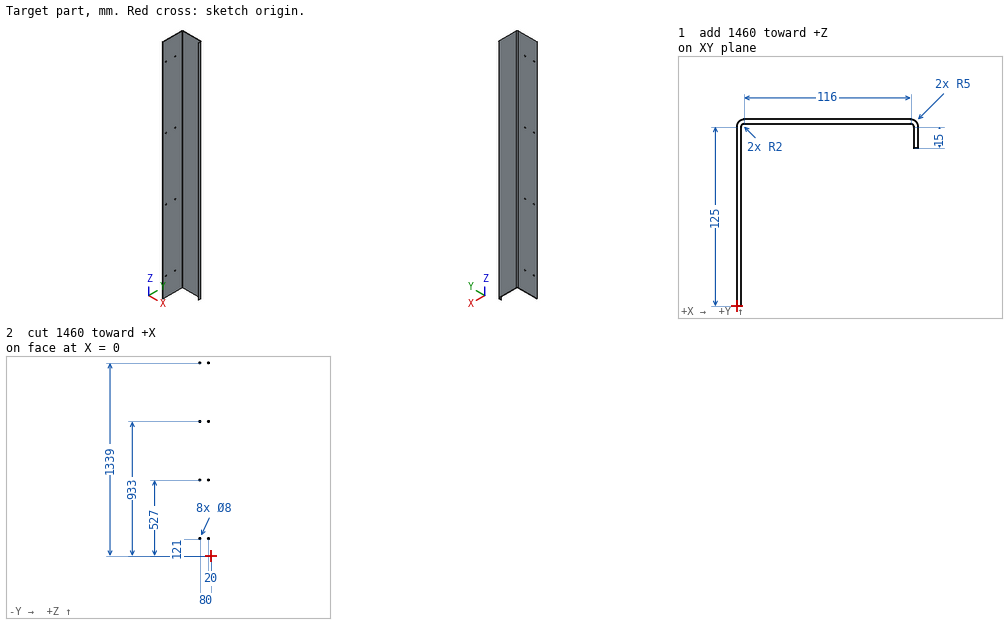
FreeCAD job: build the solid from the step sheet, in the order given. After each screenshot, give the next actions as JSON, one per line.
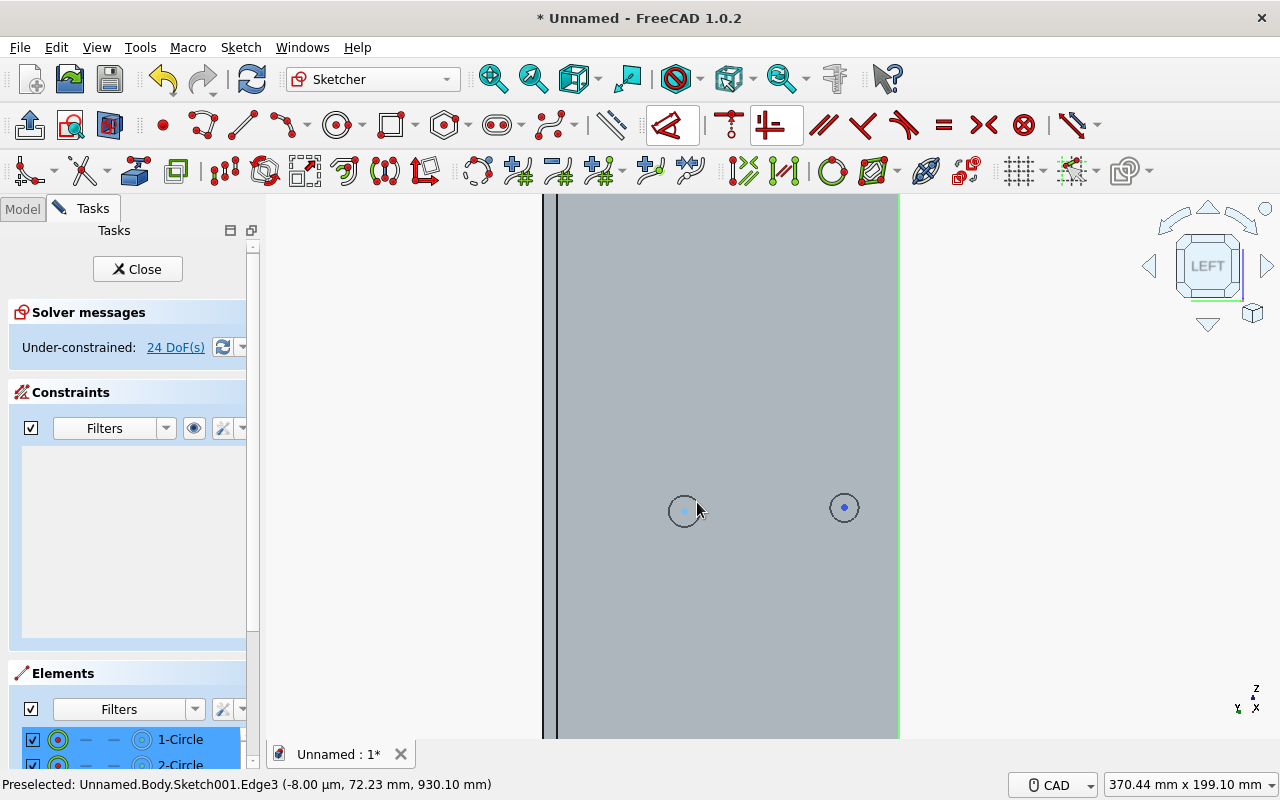
{"action": "left_click", "coordinate": [696, 500]}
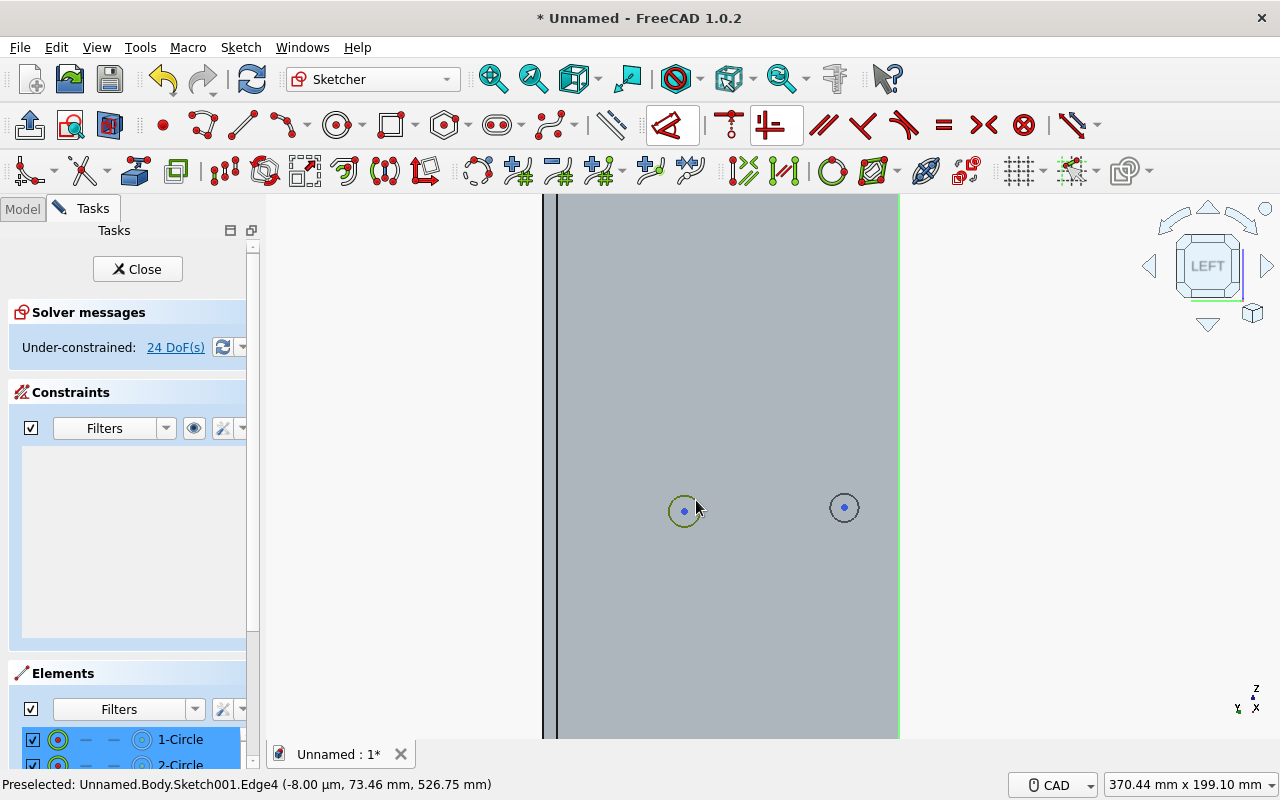
{"action": "scroll", "coordinate": [697, 502], "scroll_direction": "down", "scroll_amount": 12}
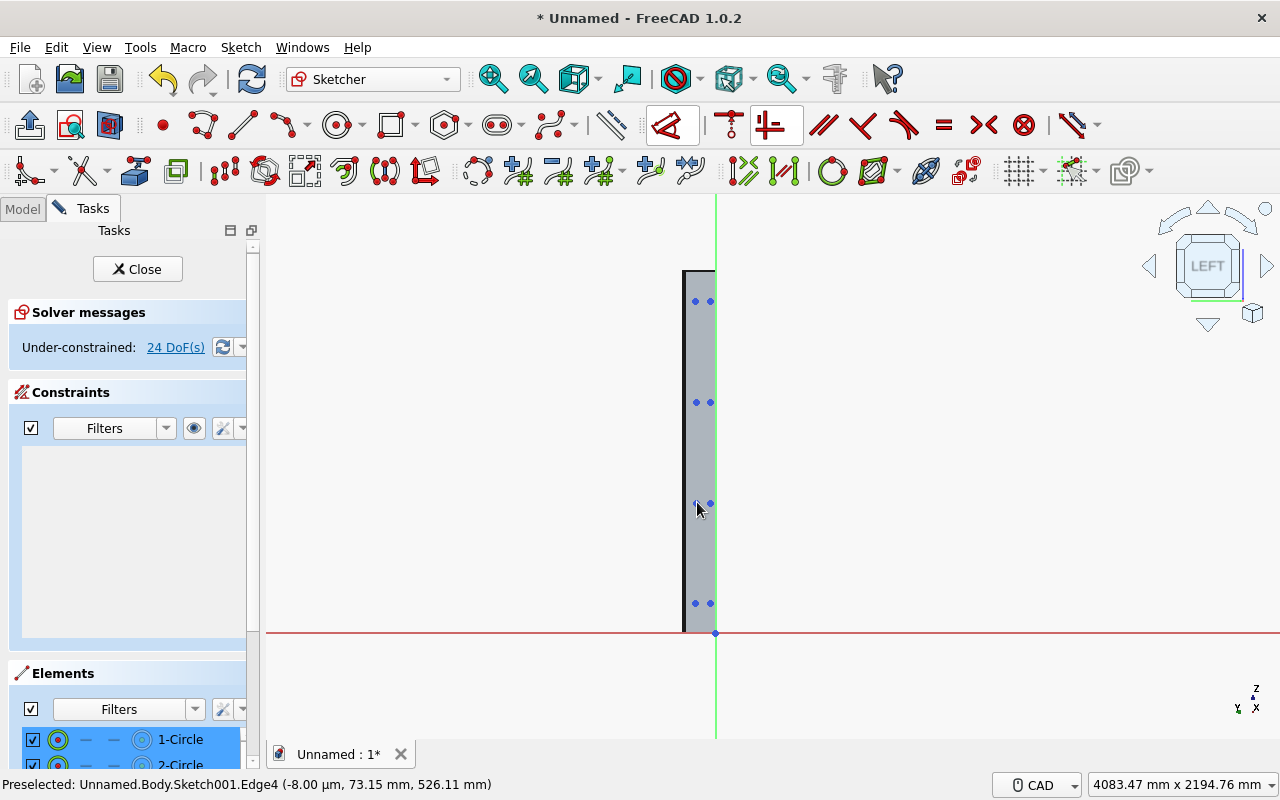
{"action": "scroll", "coordinate": [712, 603], "scroll_direction": "up", "scroll_amount": 12}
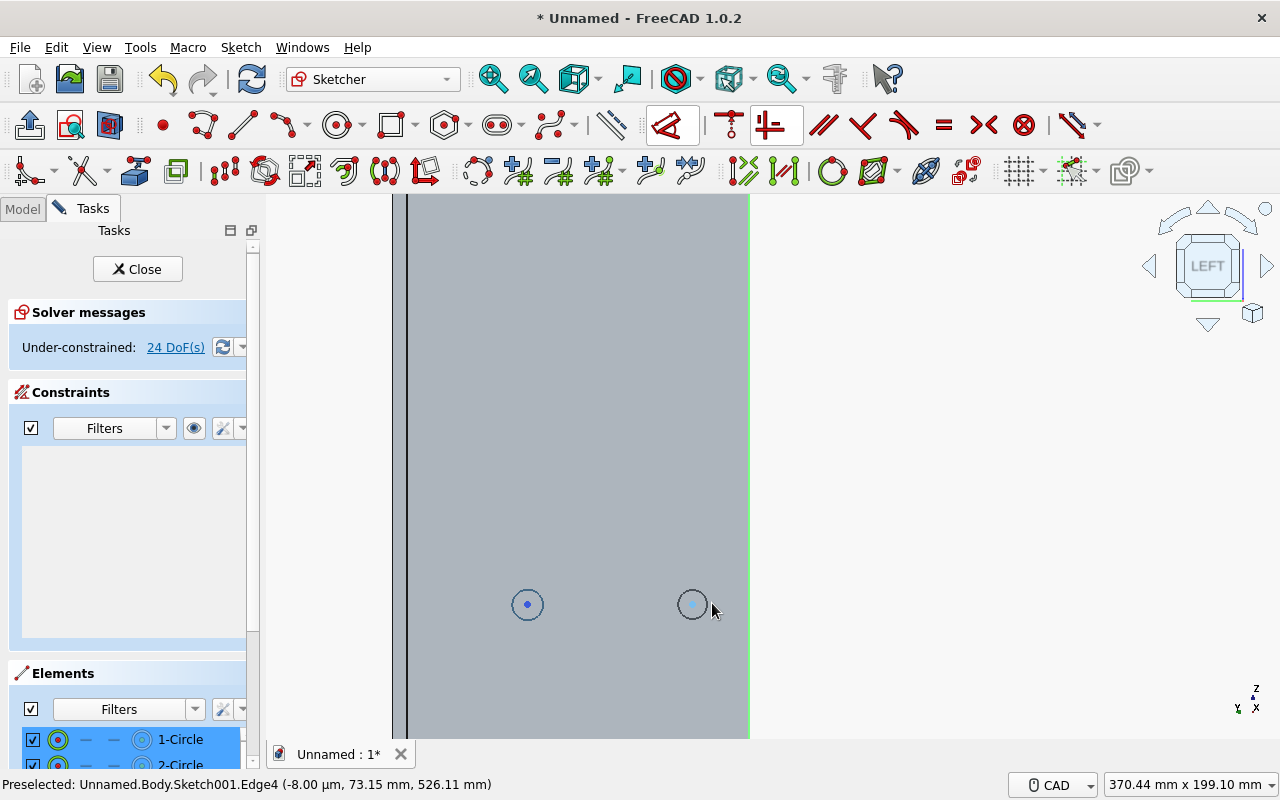
{"action": "left_click", "coordinate": [703, 594]}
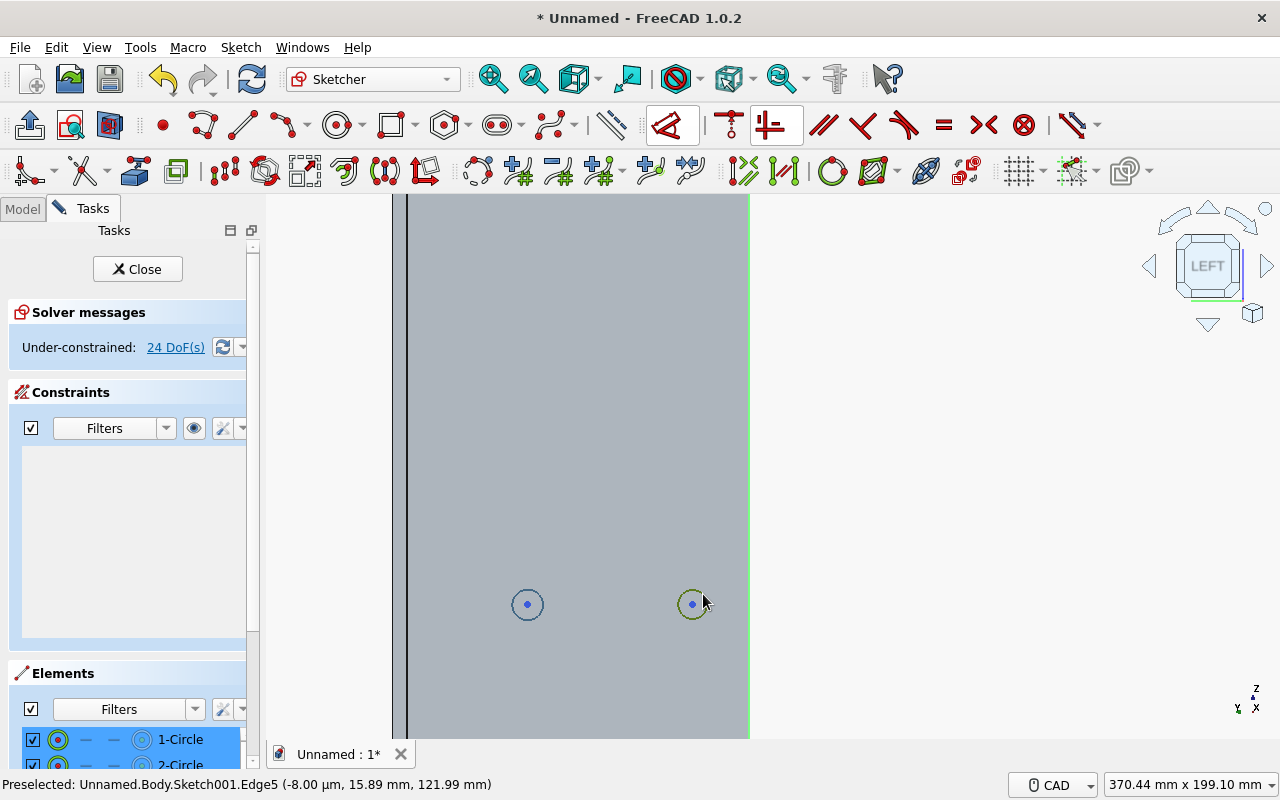
{"action": "scroll", "coordinate": [712, 603], "scroll_direction": "down", "scroll_amount": 12}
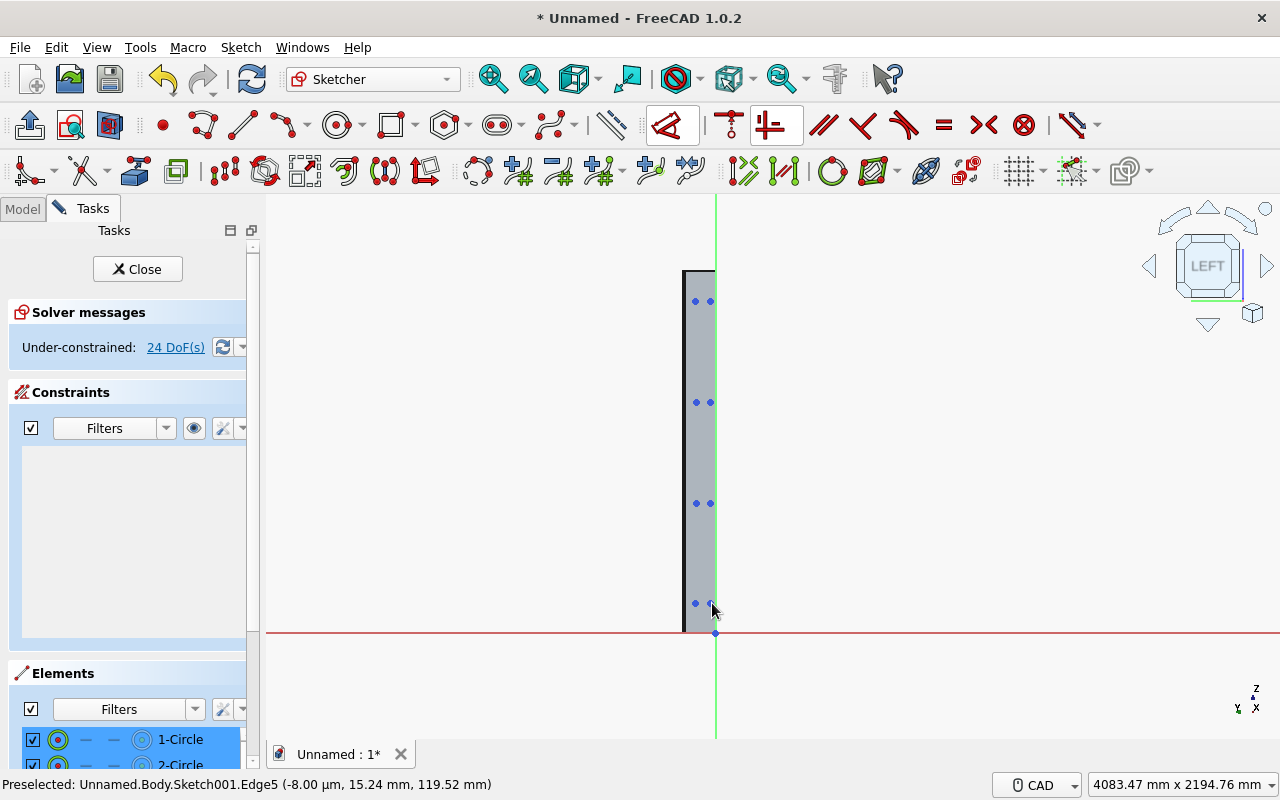
{"action": "scroll", "coordinate": [712, 300], "scroll_direction": "up", "scroll_amount": 13}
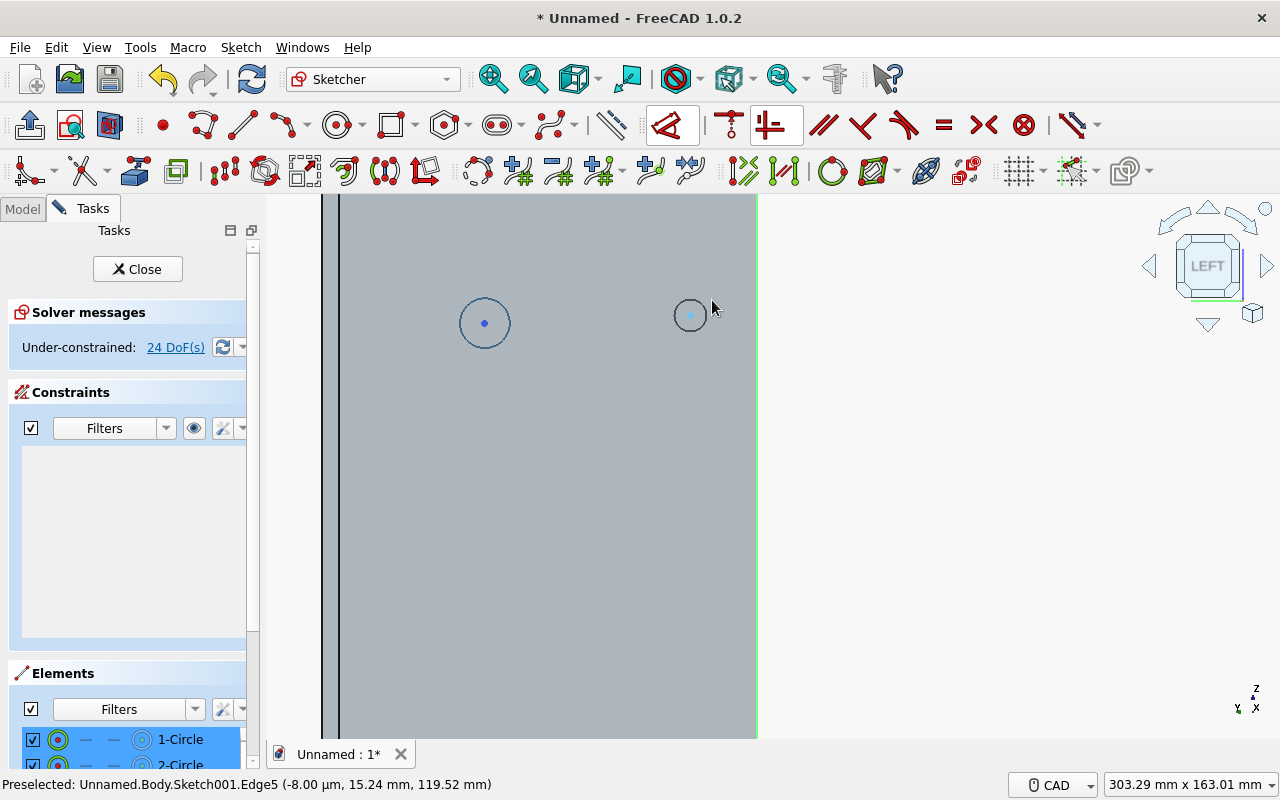
{"action": "left_click", "coordinate": [702, 304]}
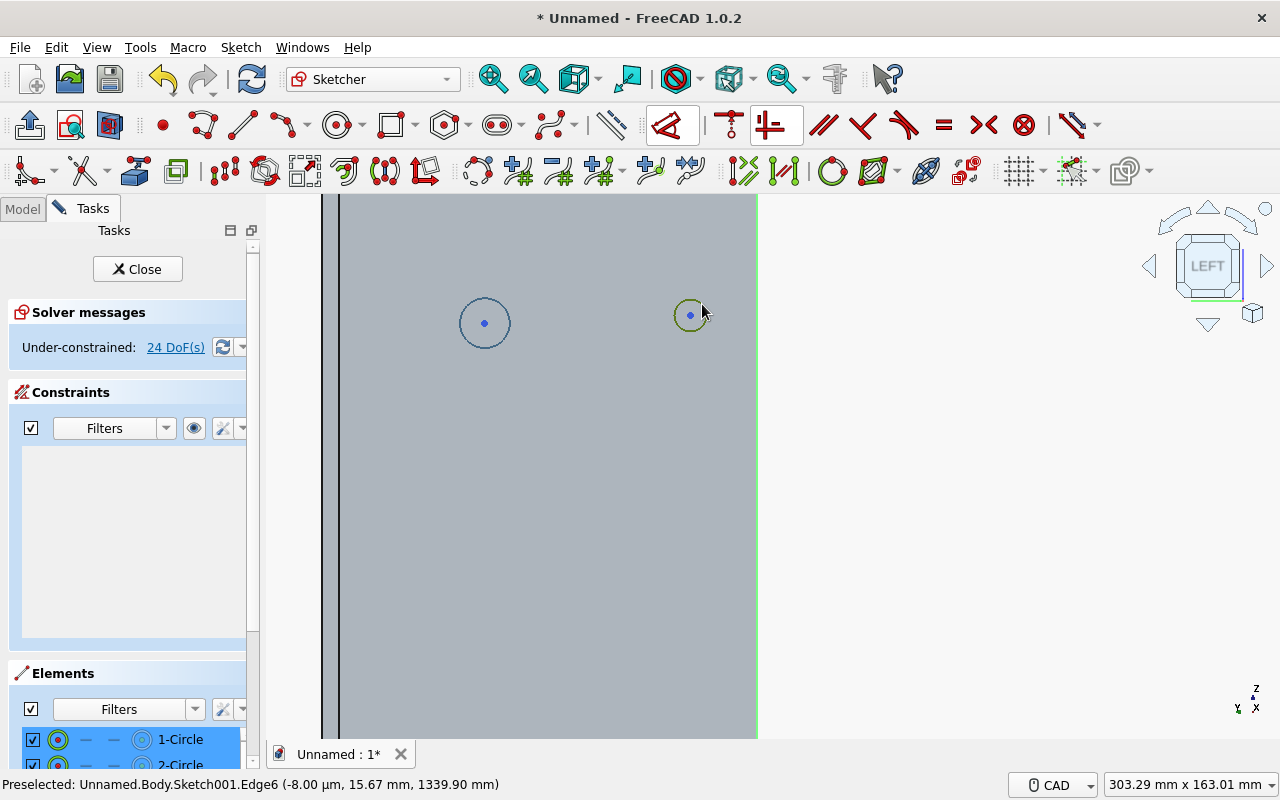
{"action": "scroll", "coordinate": [712, 300], "scroll_direction": "down", "scroll_amount": 13}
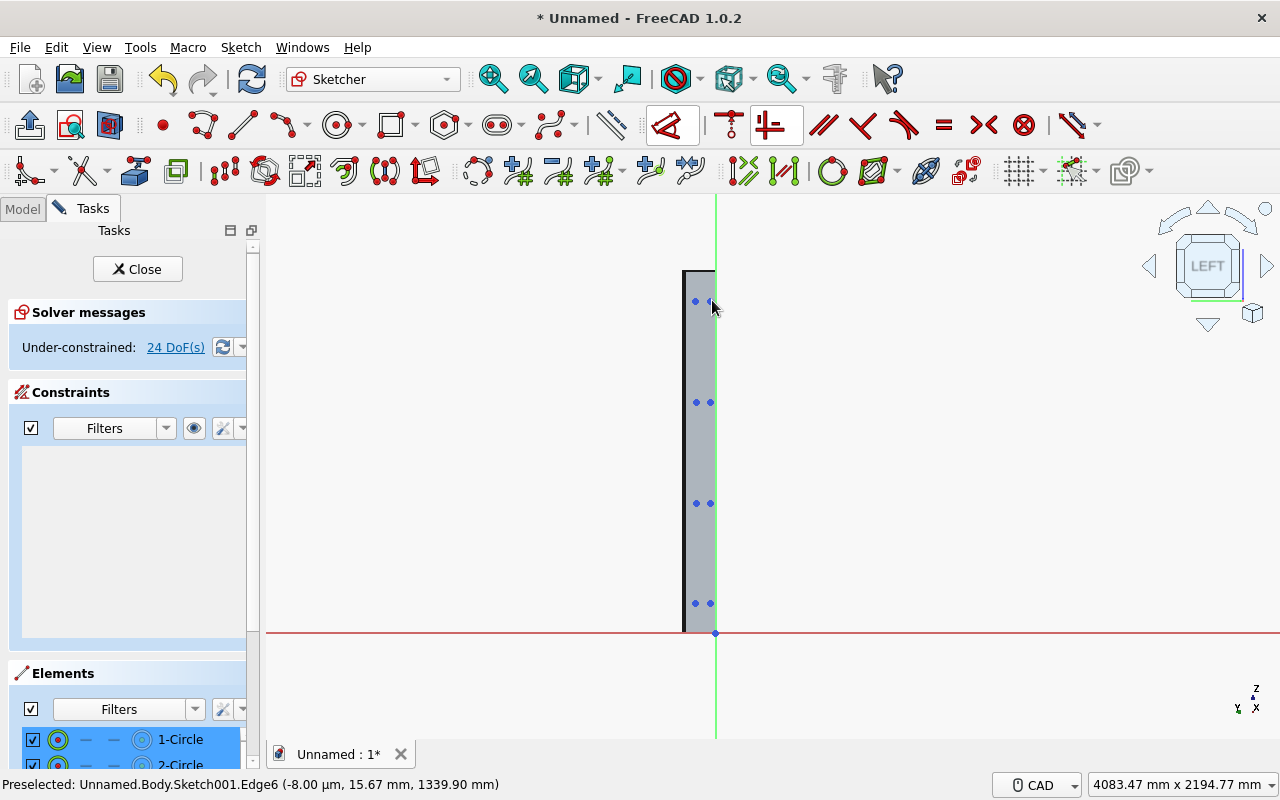
{"action": "scroll", "coordinate": [712, 401], "scroll_direction": "up", "scroll_amount": 13}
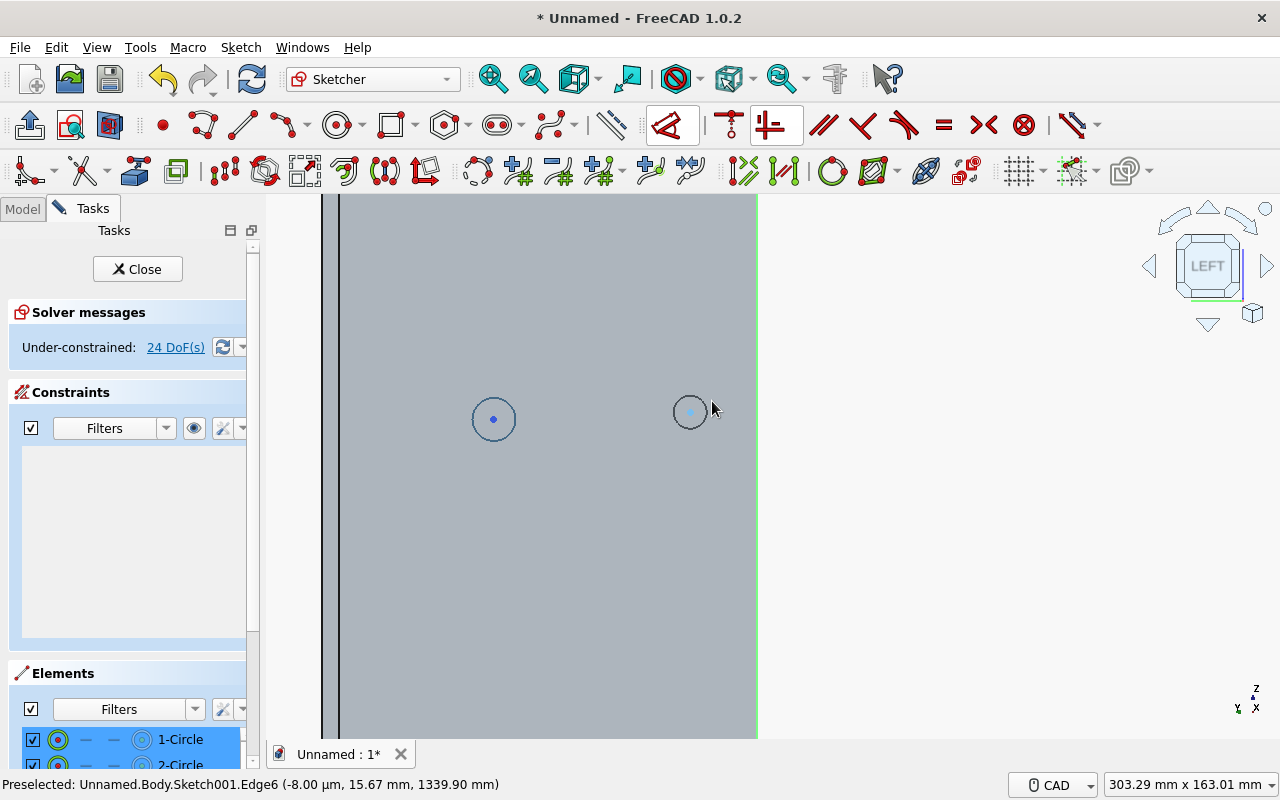
{"action": "left_click", "coordinate": [702, 401]}